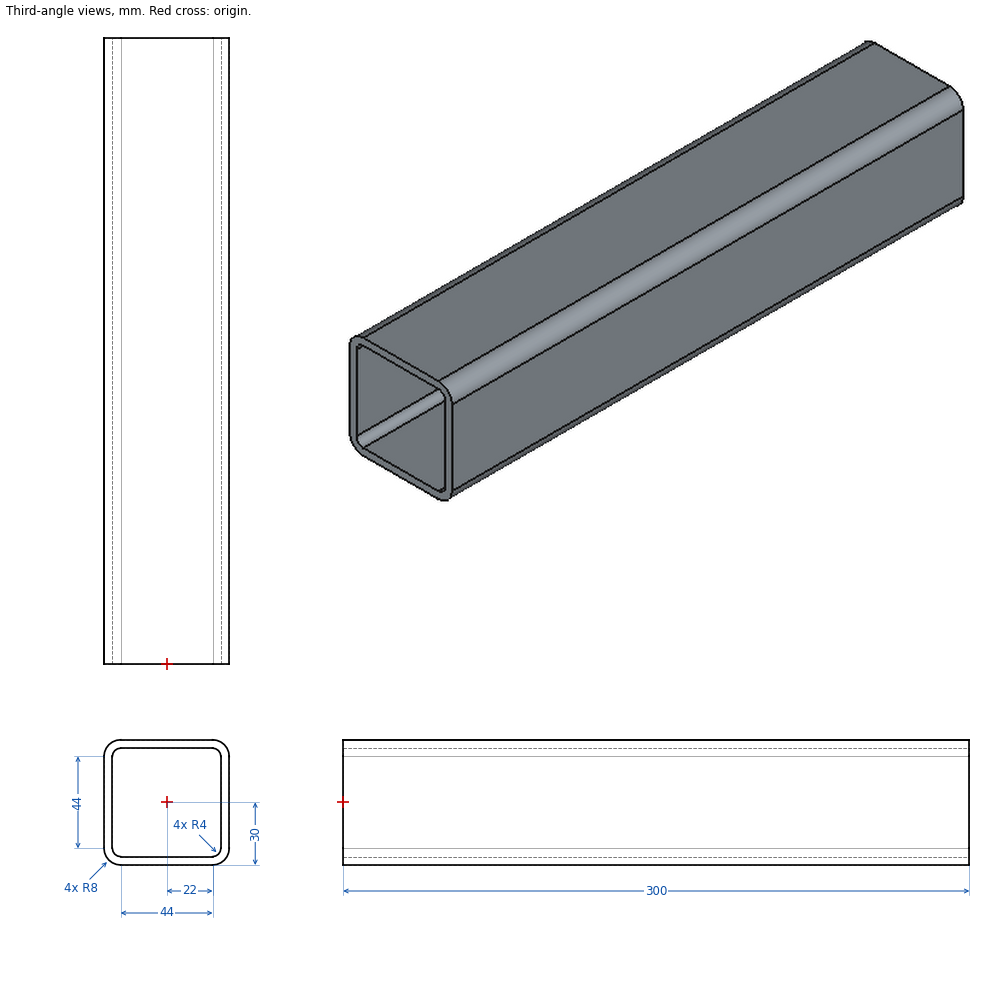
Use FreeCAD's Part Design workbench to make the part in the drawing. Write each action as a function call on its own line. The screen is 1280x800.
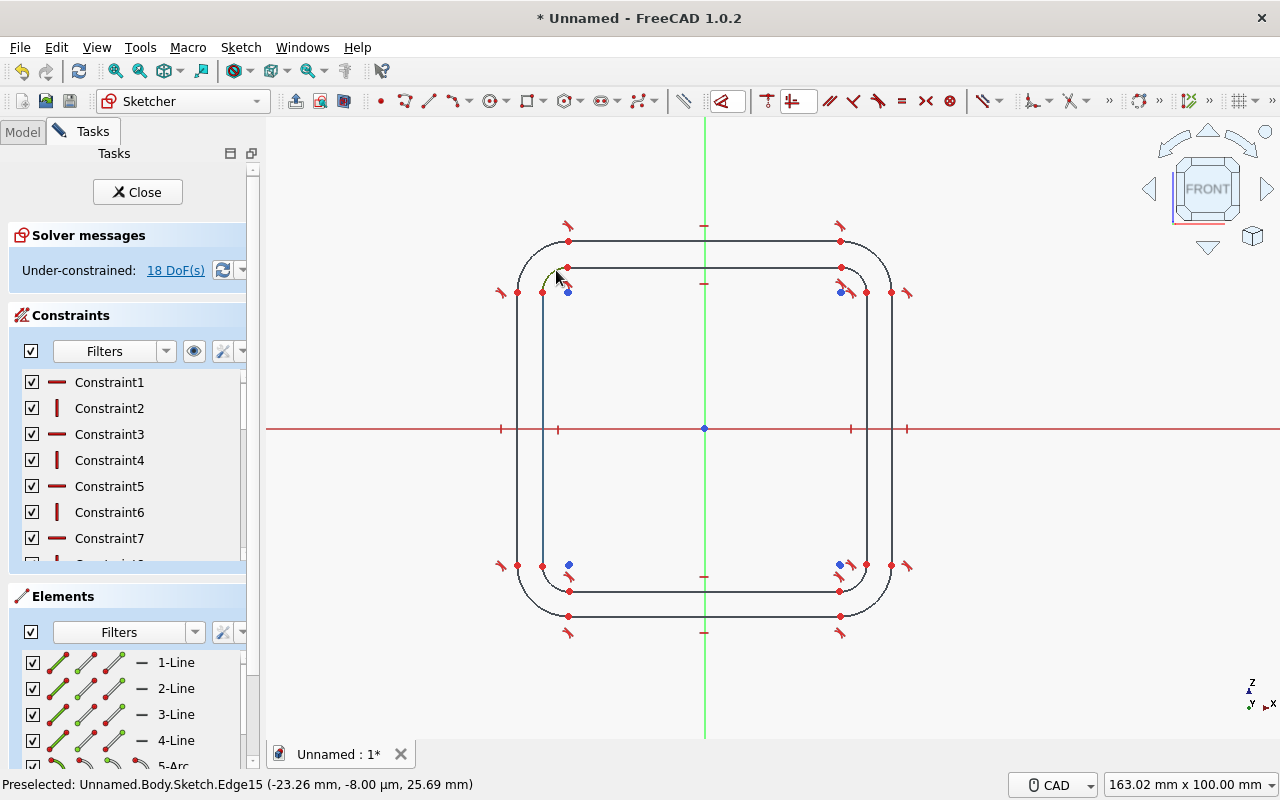
key(t)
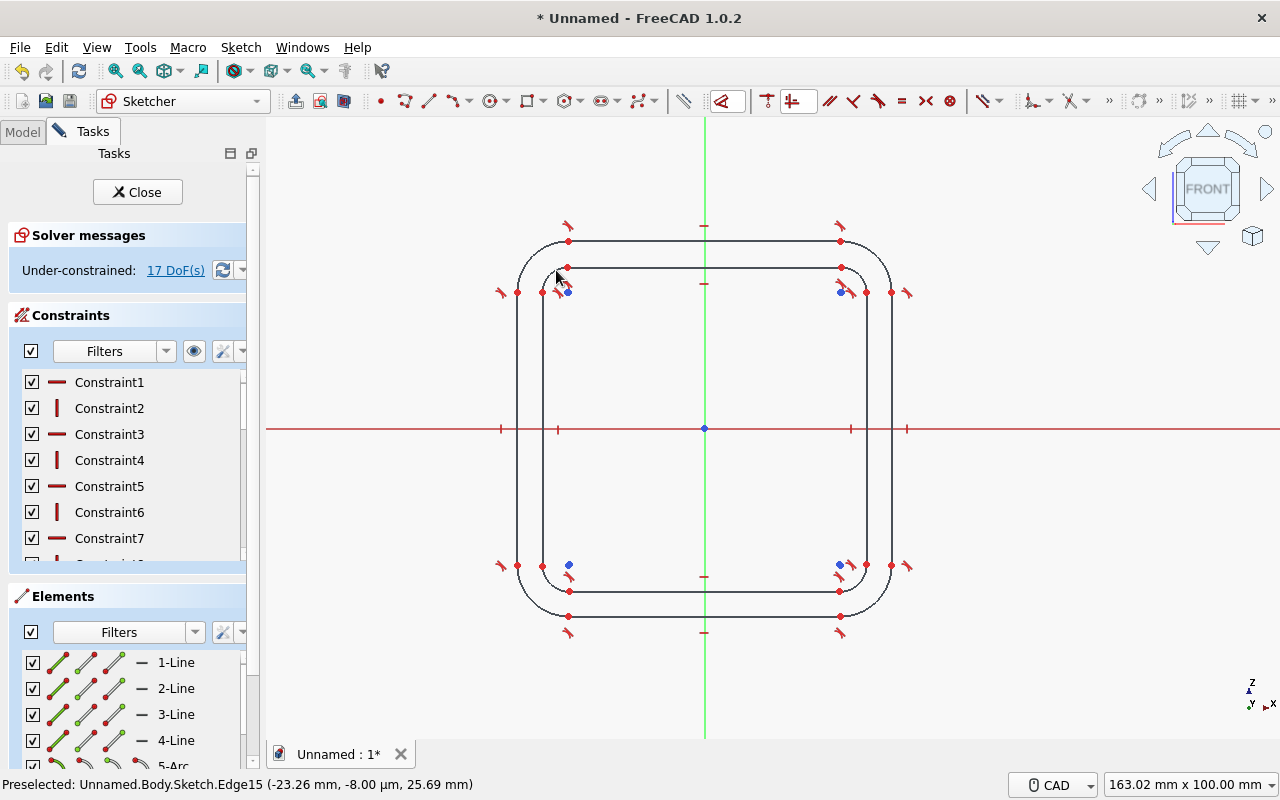
click(543, 375)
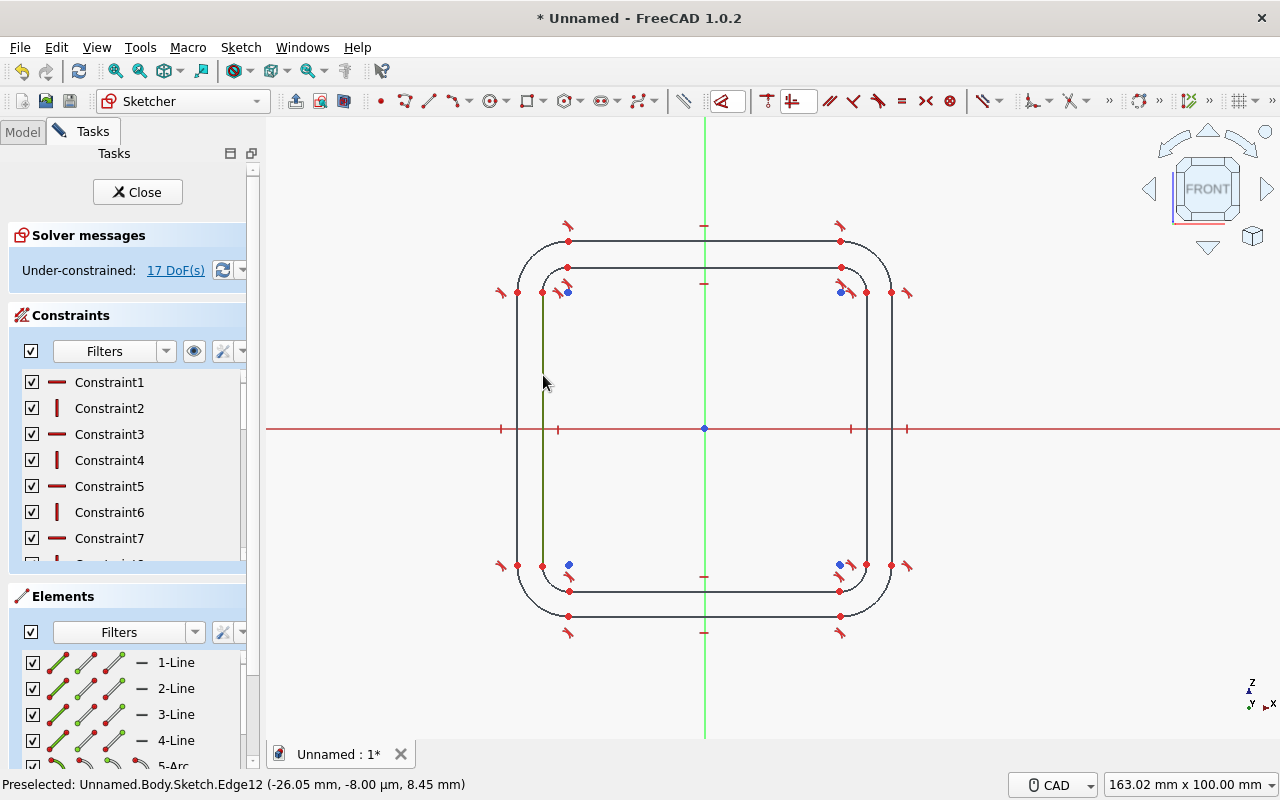
click(546, 578)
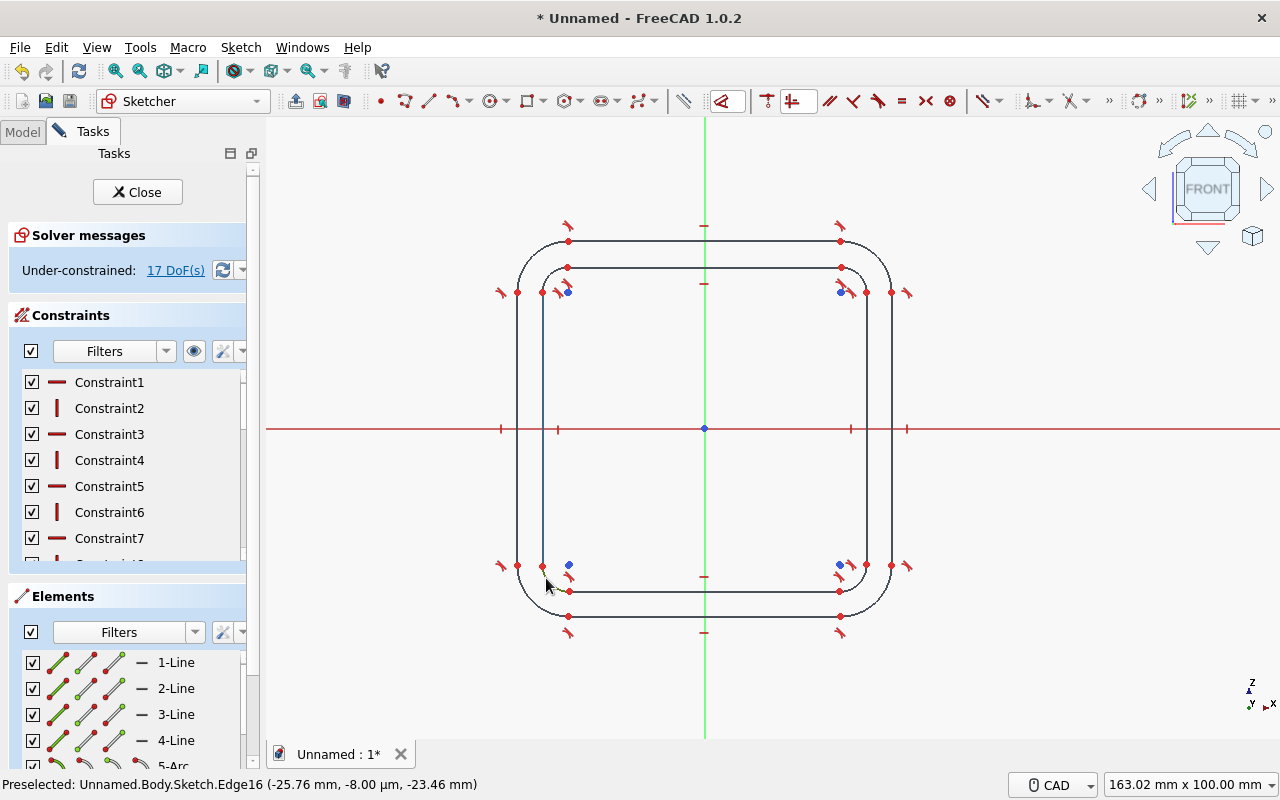
click(878, 102)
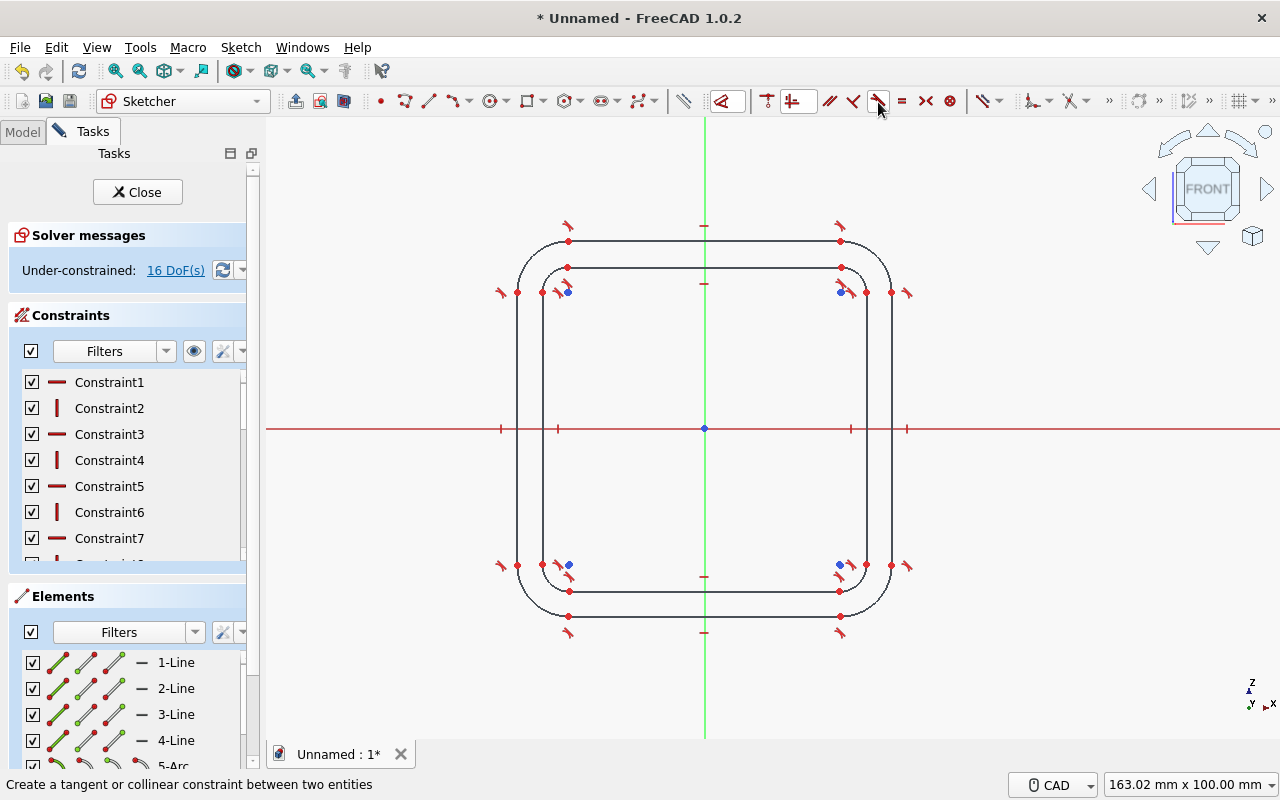
click(864, 611)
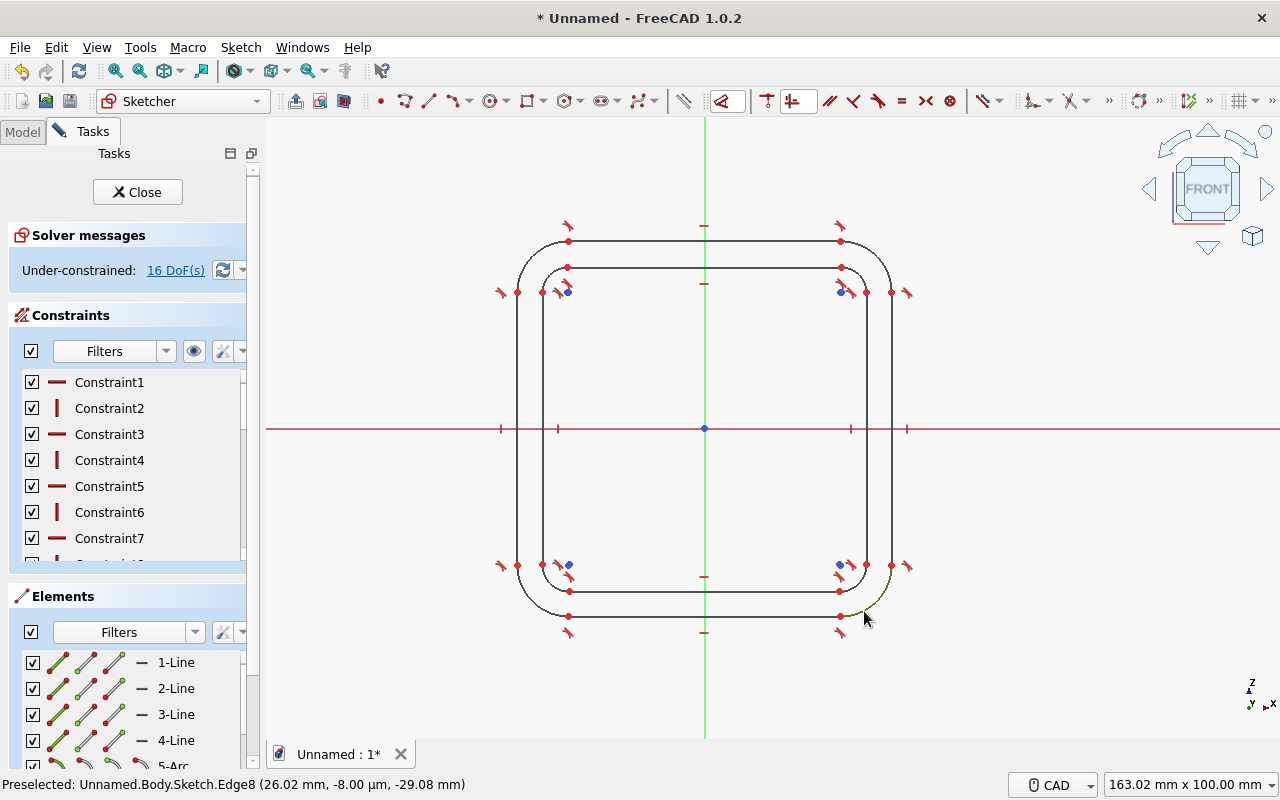
click(852, 589)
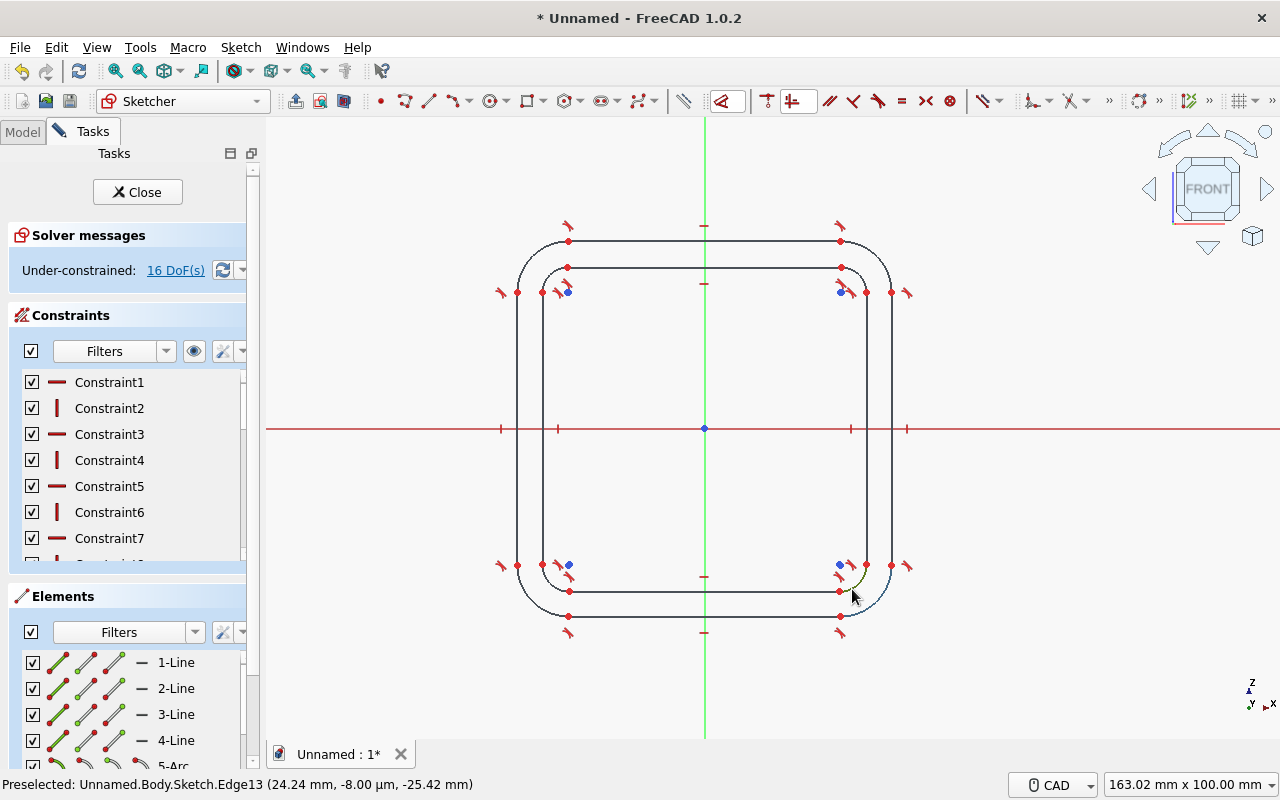
click(768, 102)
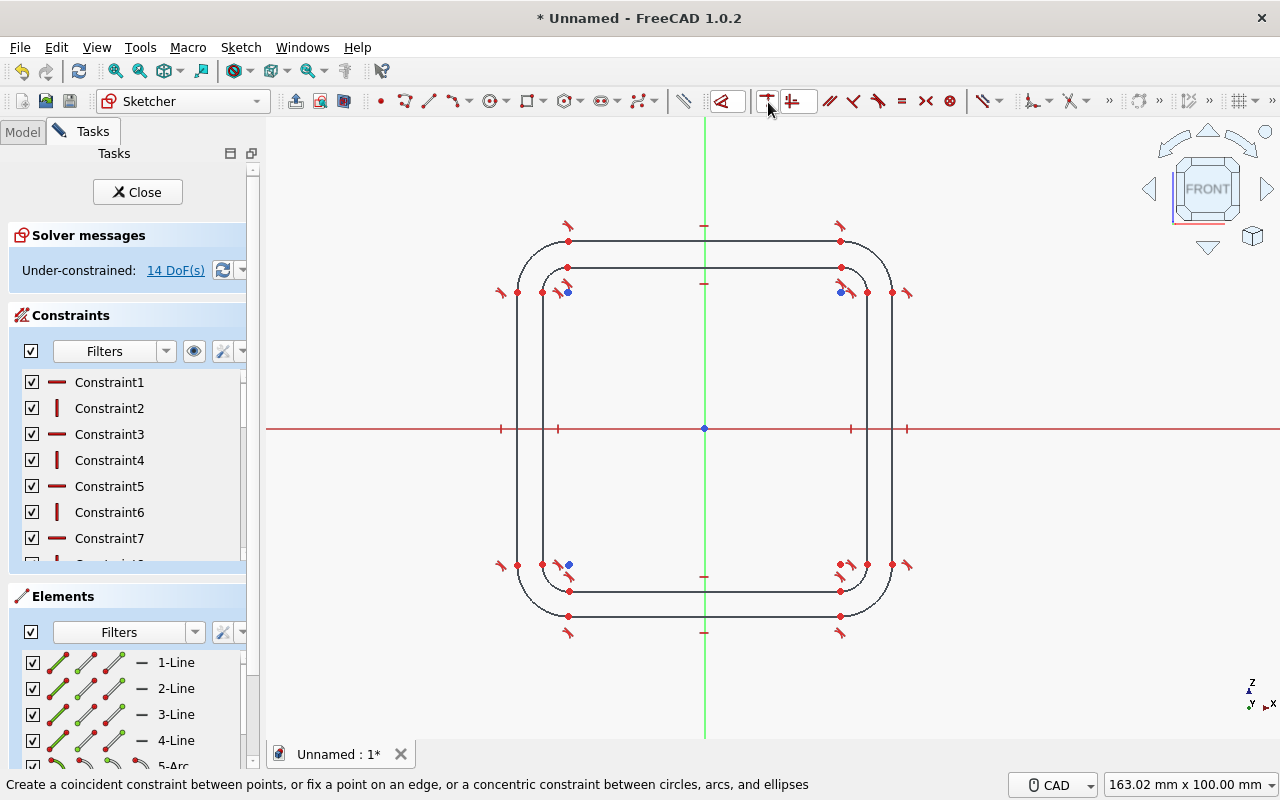
click(886, 269)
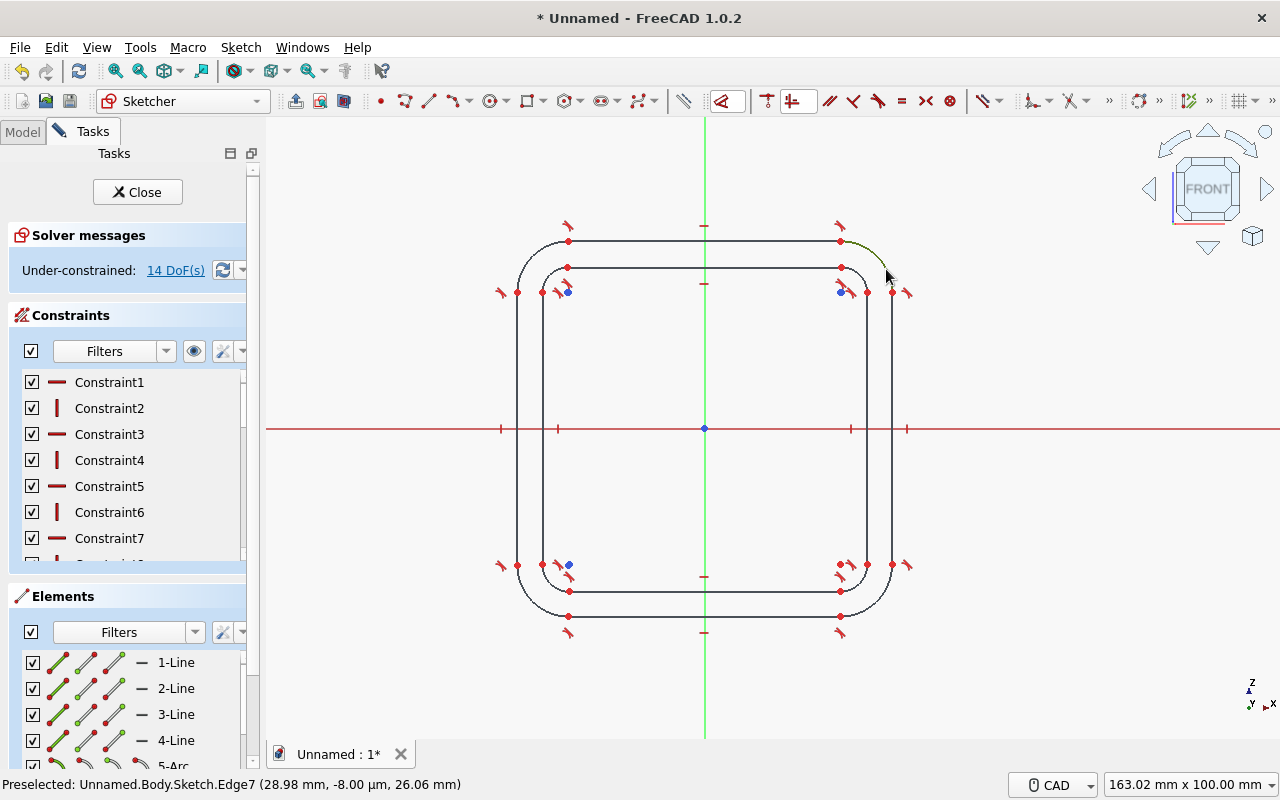
click(864, 281)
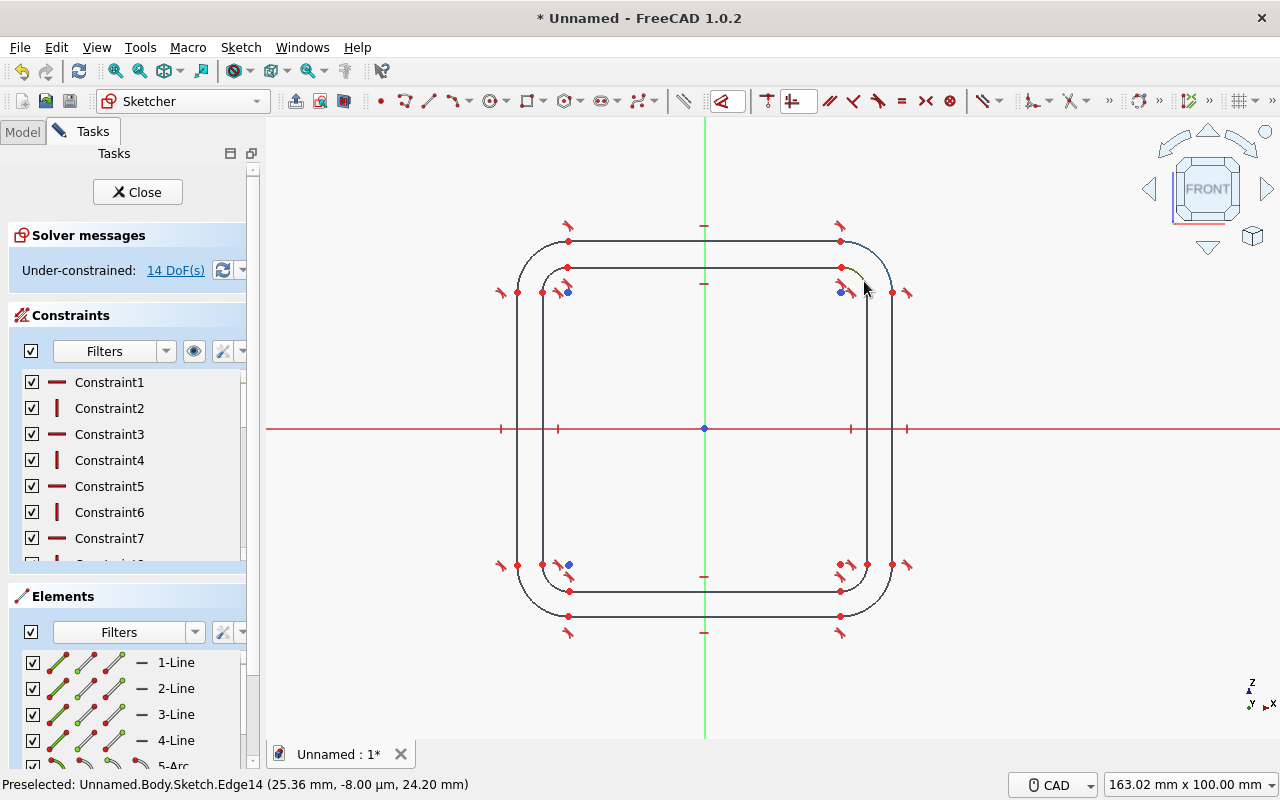
key(c)